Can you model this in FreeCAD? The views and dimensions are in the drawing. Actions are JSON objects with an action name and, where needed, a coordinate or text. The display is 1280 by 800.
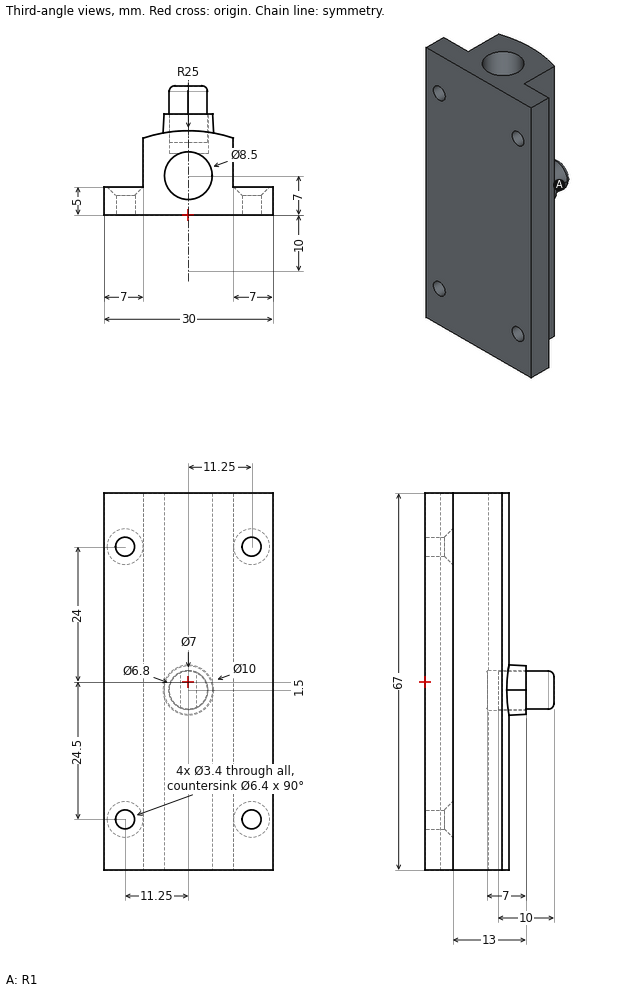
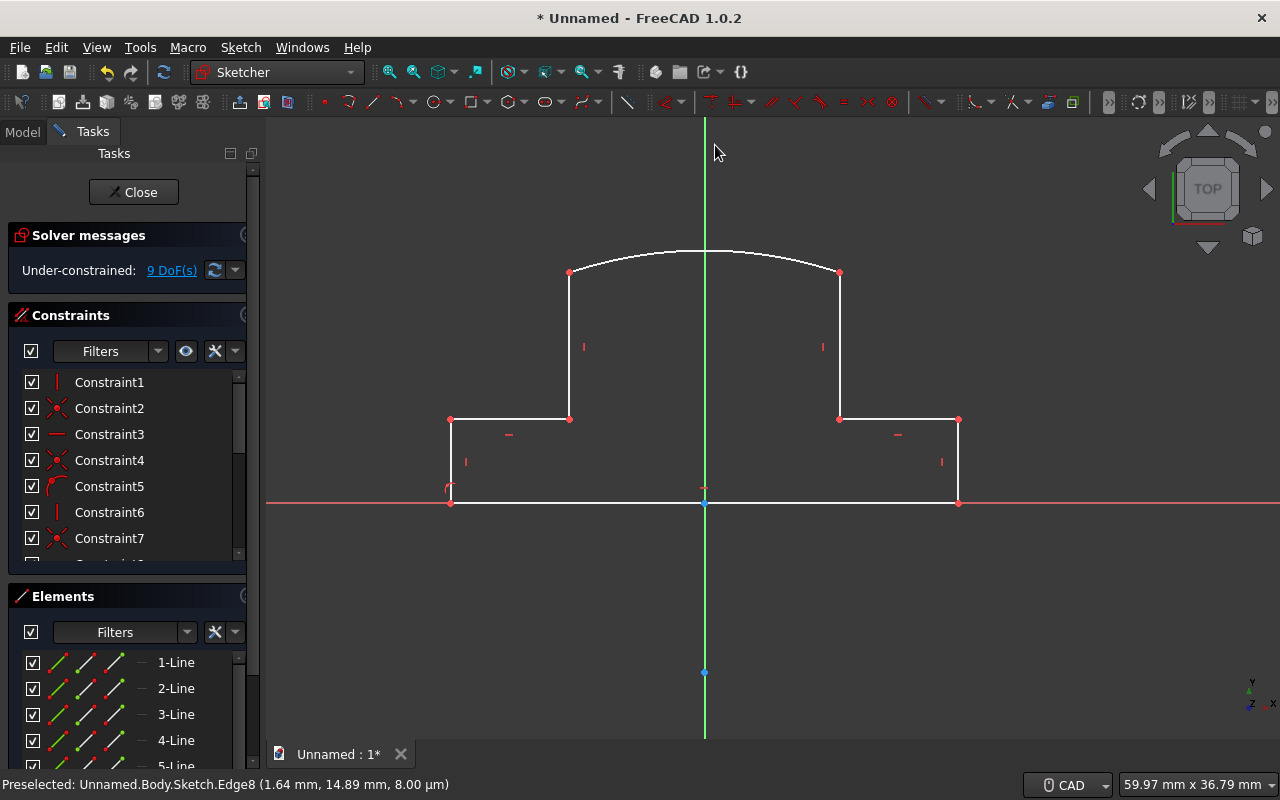
{"action": "left_click", "coordinate": [704, 673]}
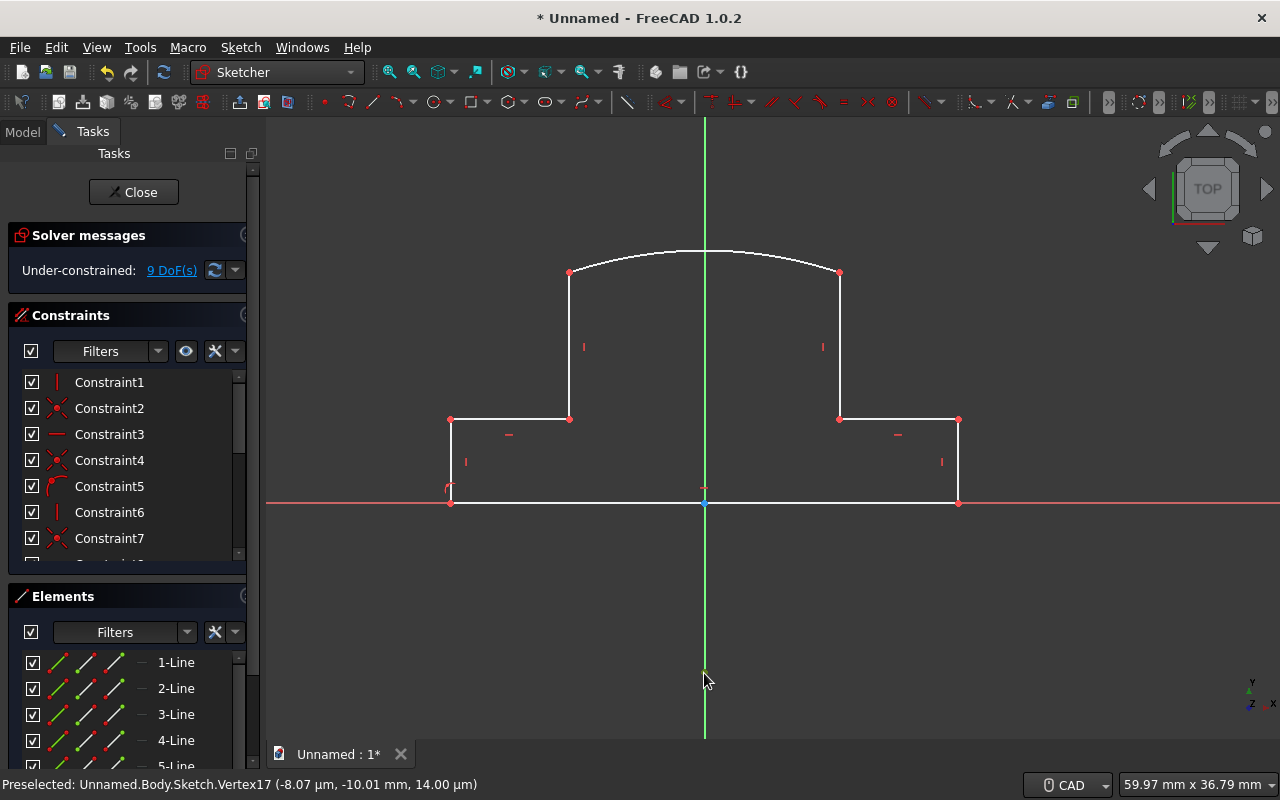
{"action": "left_click", "coordinate": [705, 630]}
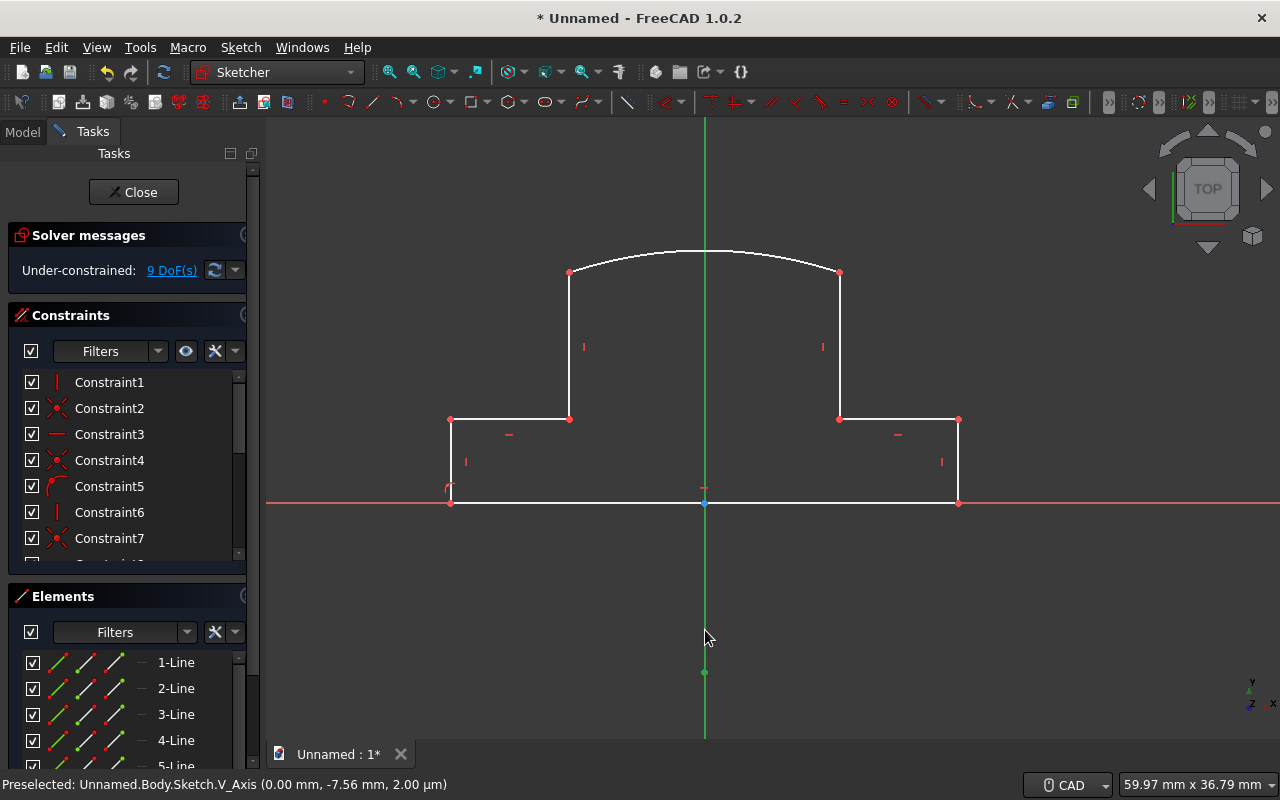
{"action": "left_click", "coordinate": [712, 102]}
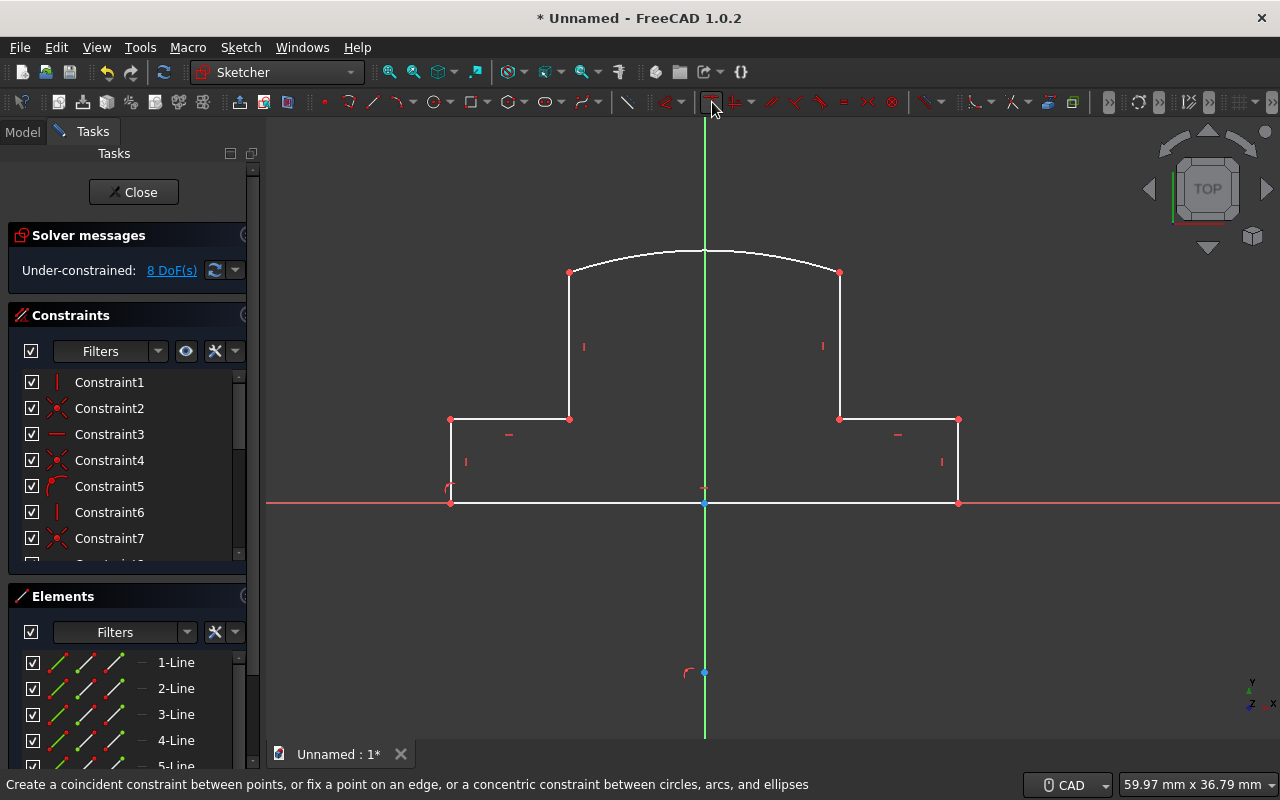
{"action": "left_click", "coordinate": [451, 419]}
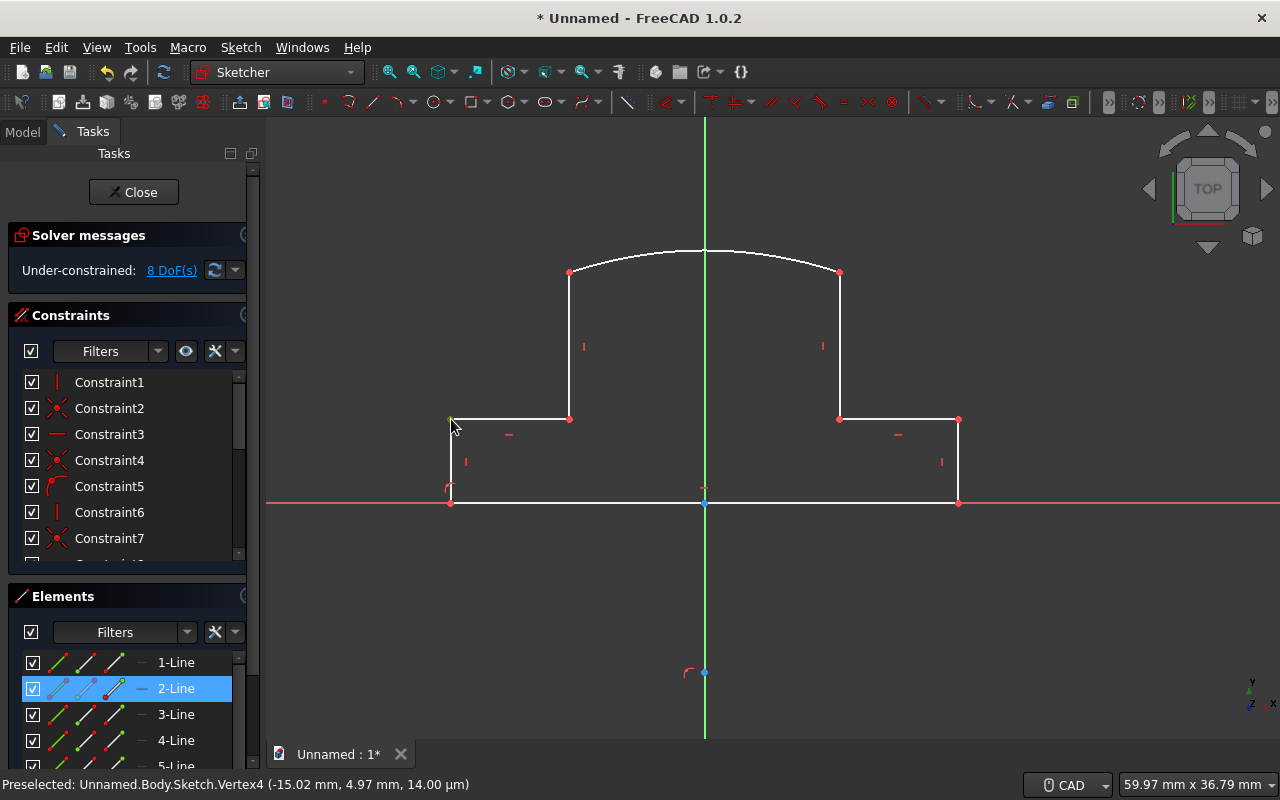
{"action": "left_click", "coordinate": [958, 419]}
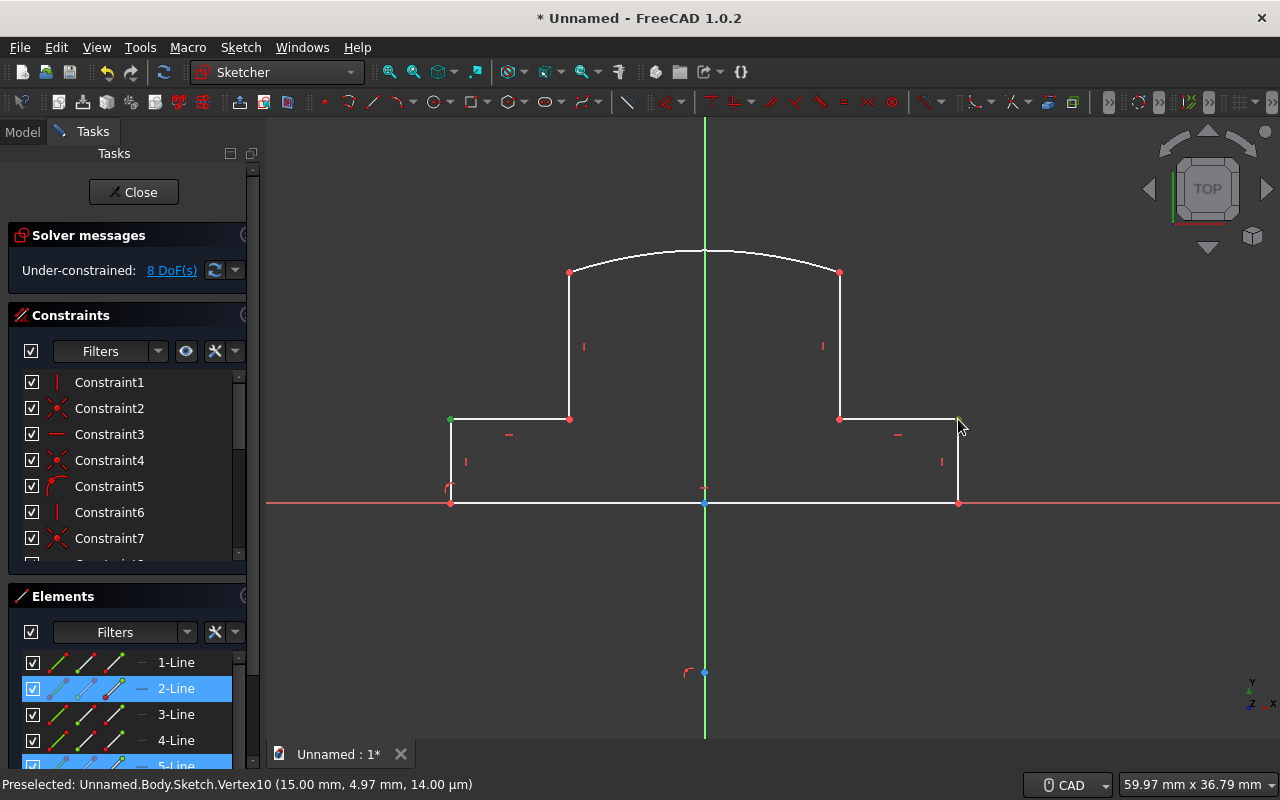
{"action": "left_click", "coordinate": [705, 630]}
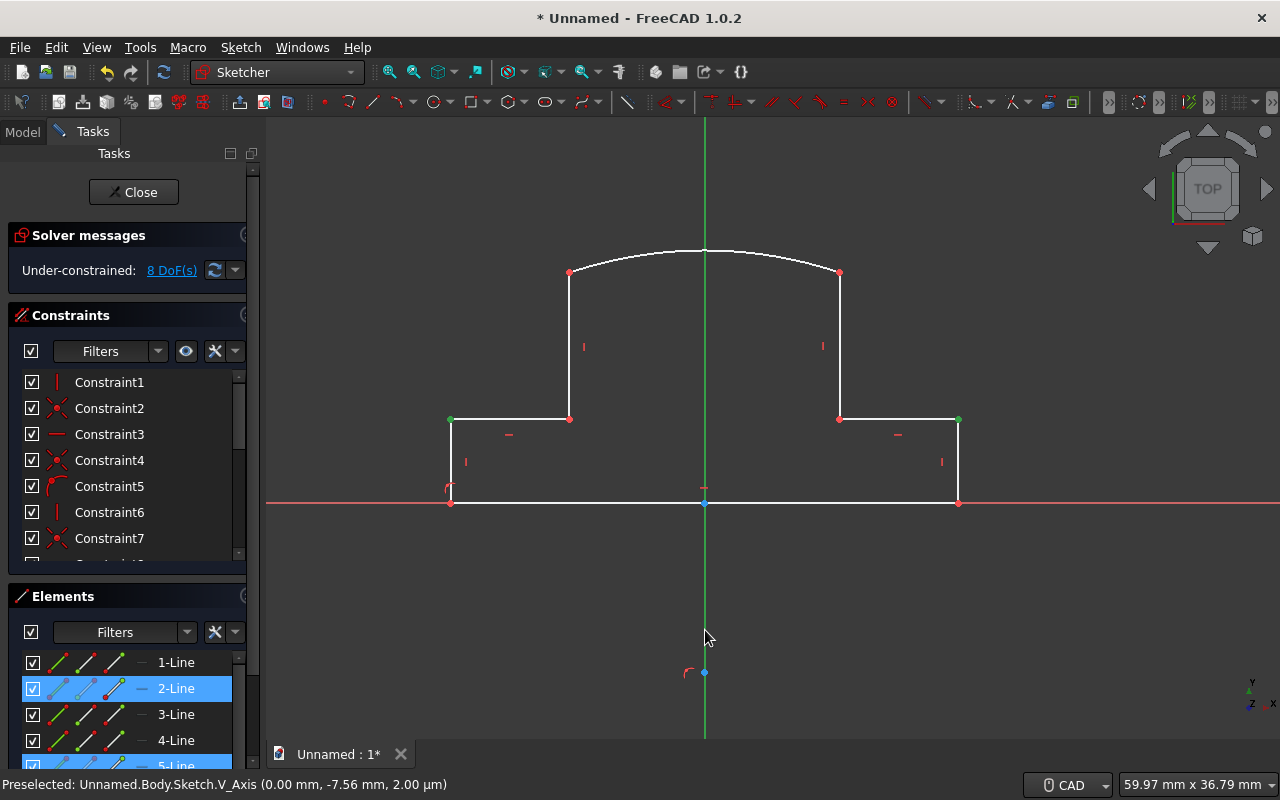
{"action": "key", "text": "s"}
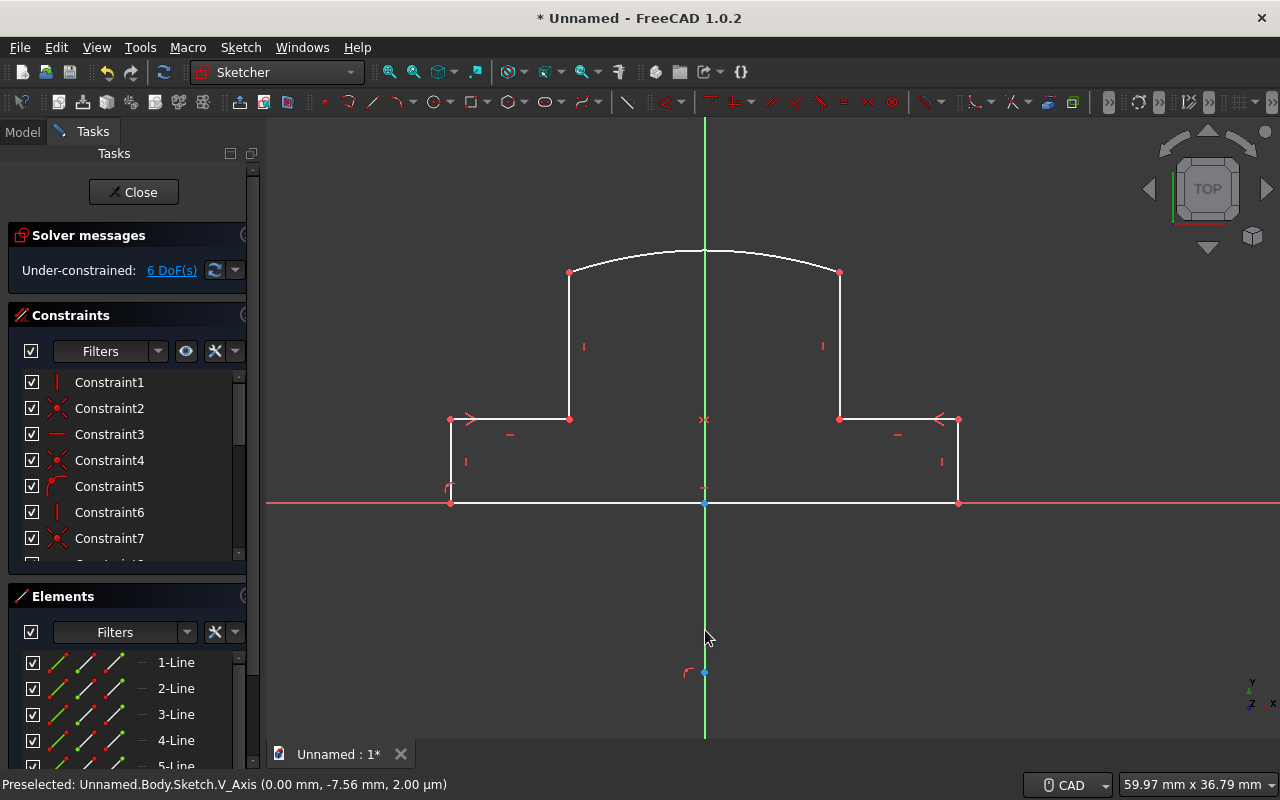
{"action": "left_click", "coordinate": [759, 254]}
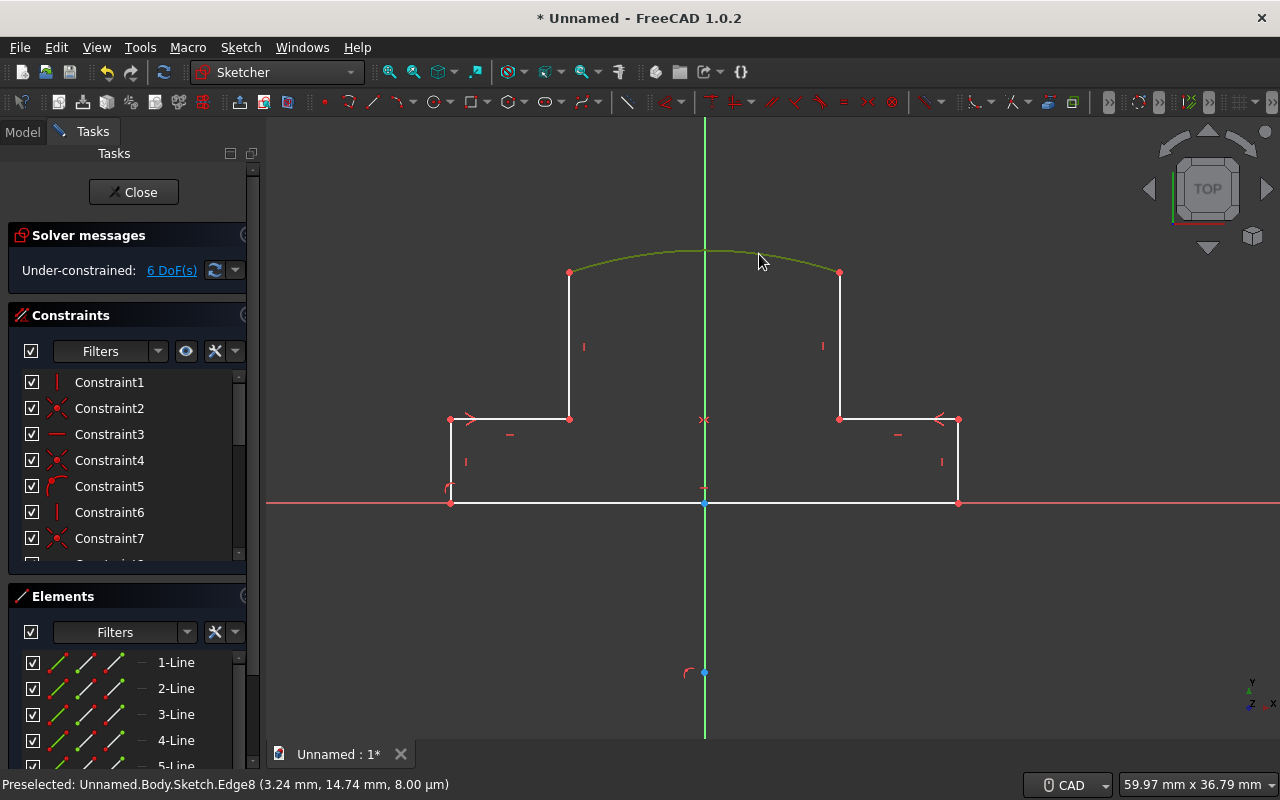
{"action": "key", "text": "k r"}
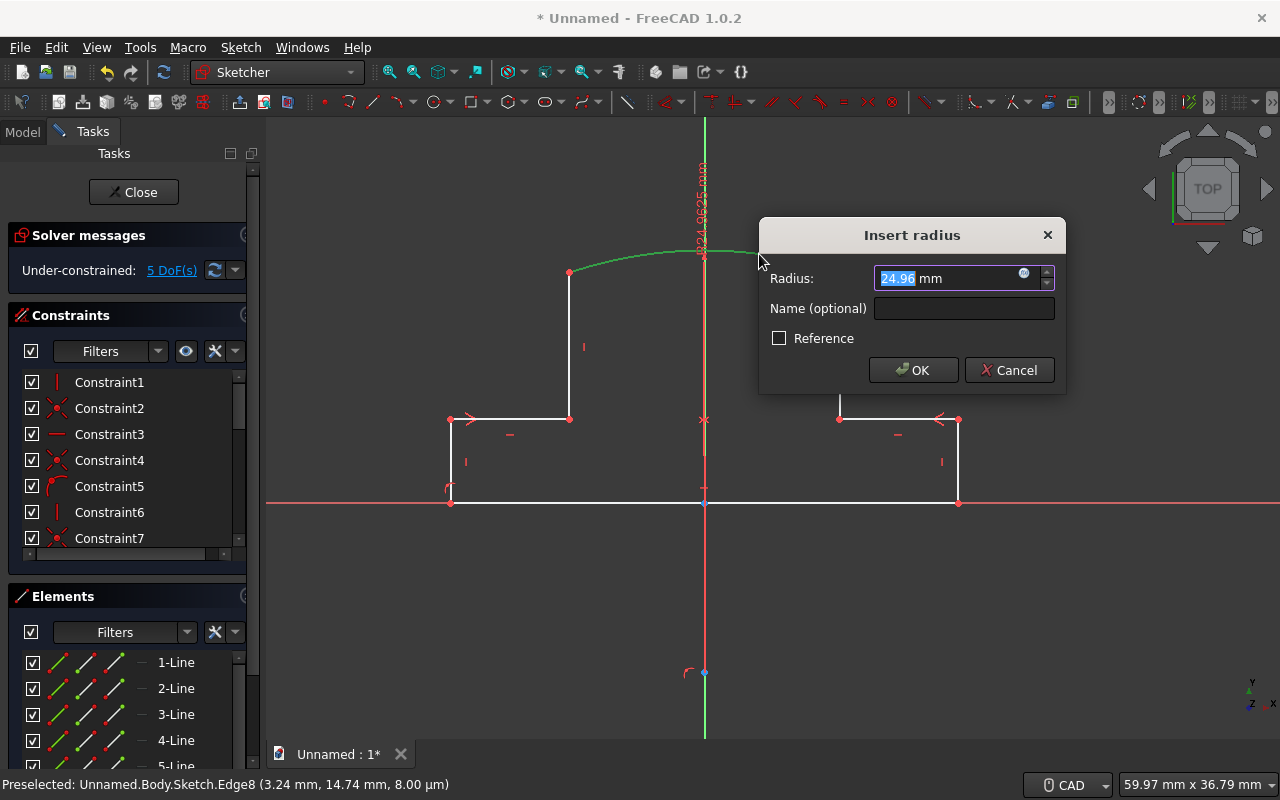
{"action": "type", "text": "25"}
{"action": "key", "text": "Return"}